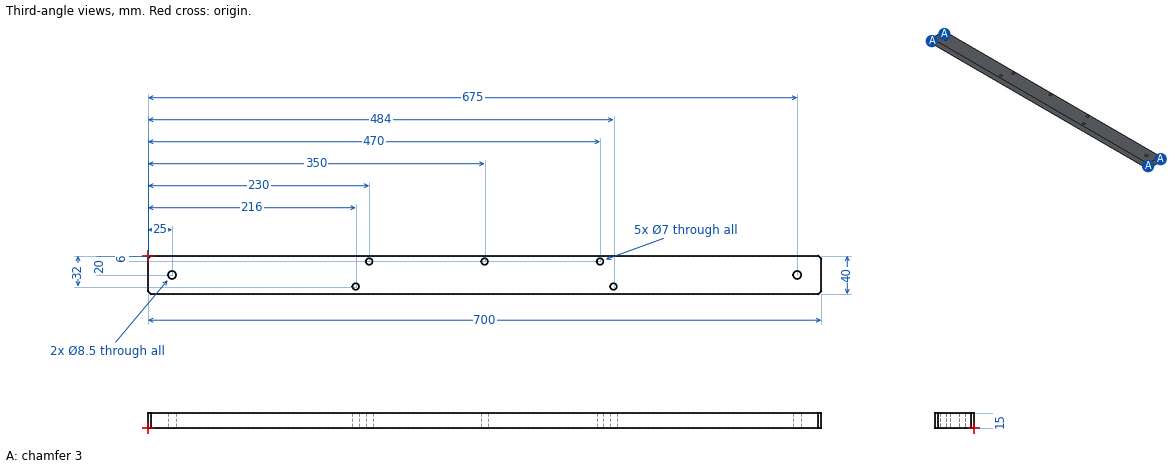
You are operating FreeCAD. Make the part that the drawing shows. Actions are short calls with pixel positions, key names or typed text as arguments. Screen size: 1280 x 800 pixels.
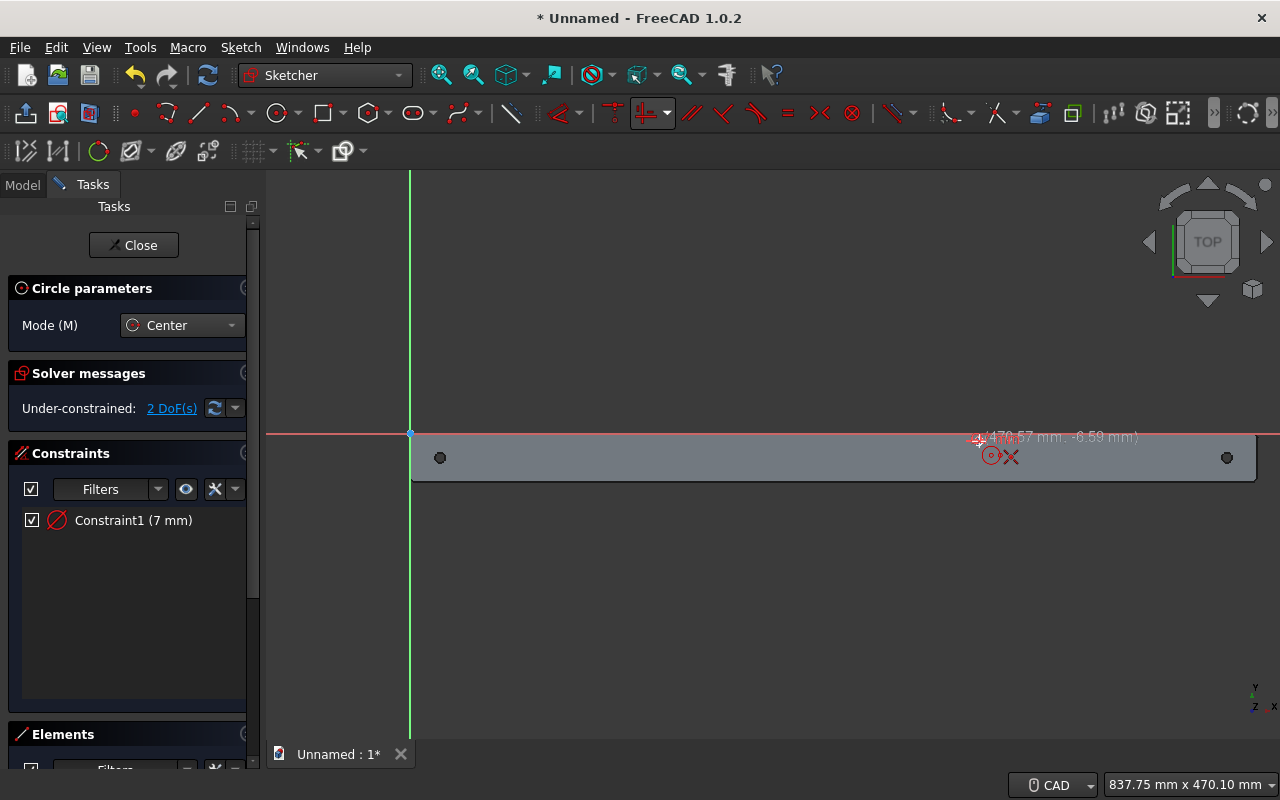
scroll(834, 441, up, 9)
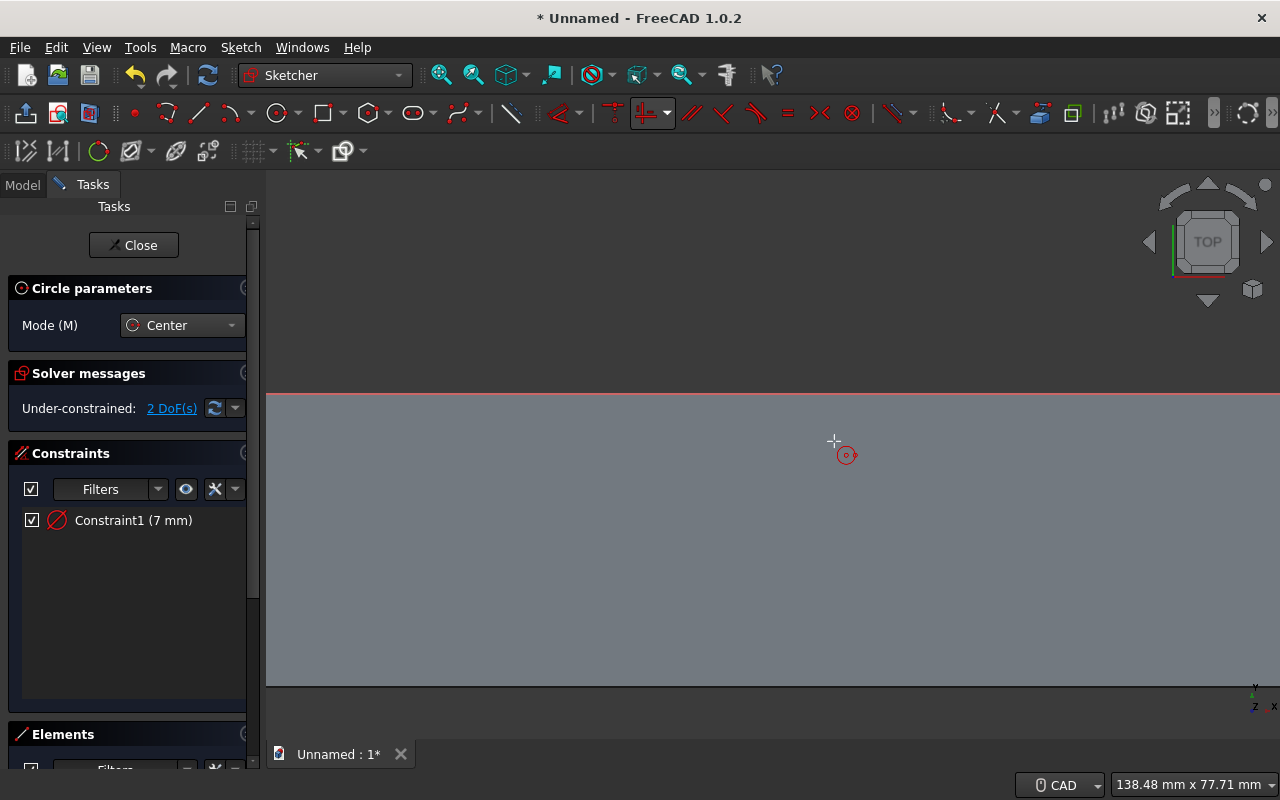
click(829, 438)
move(847, 420)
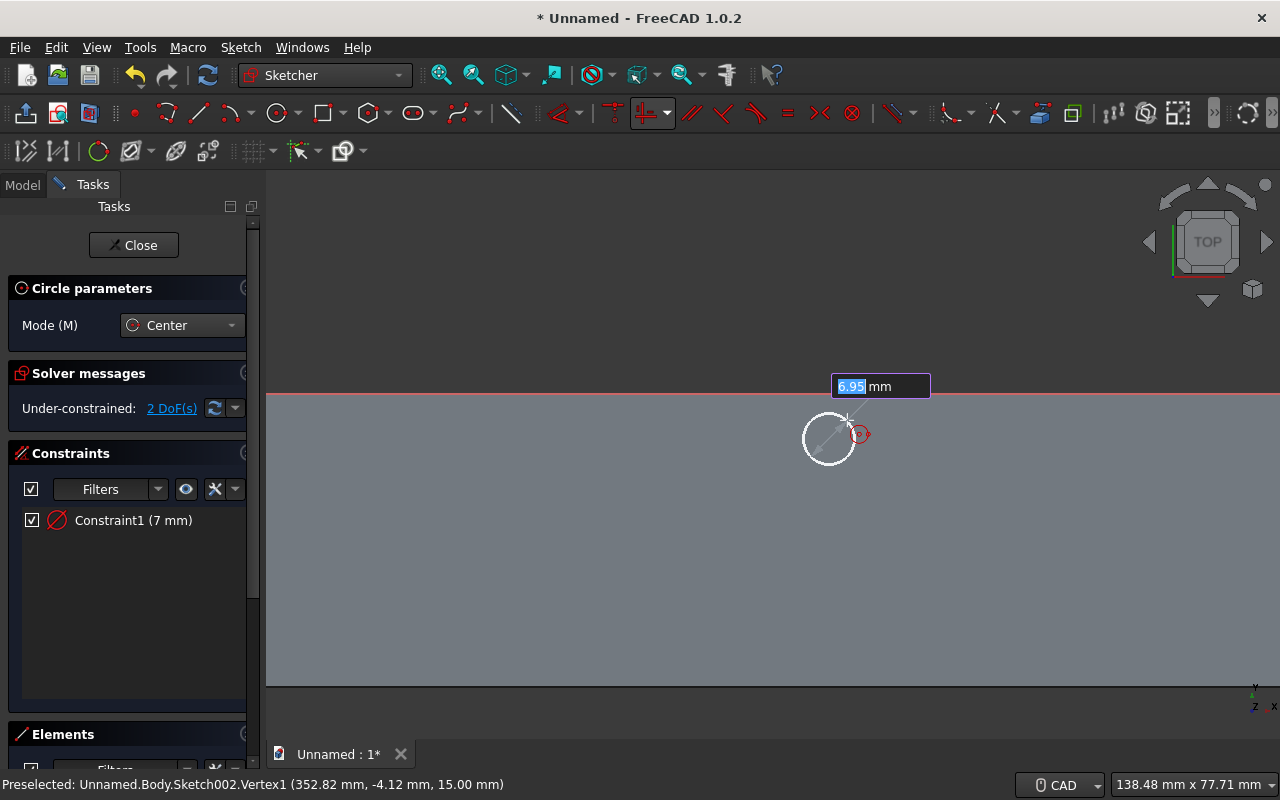
text(7)
key(Return)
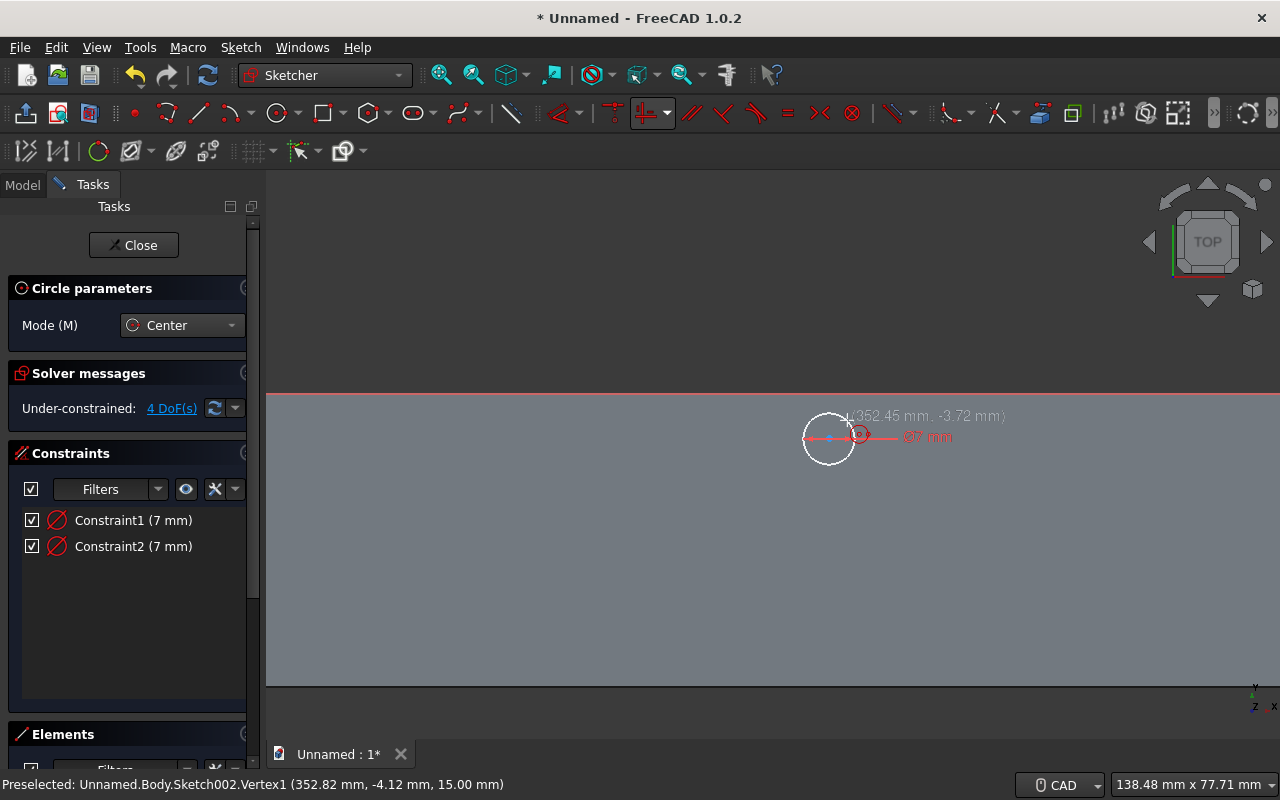
scroll(834, 441, down, 9)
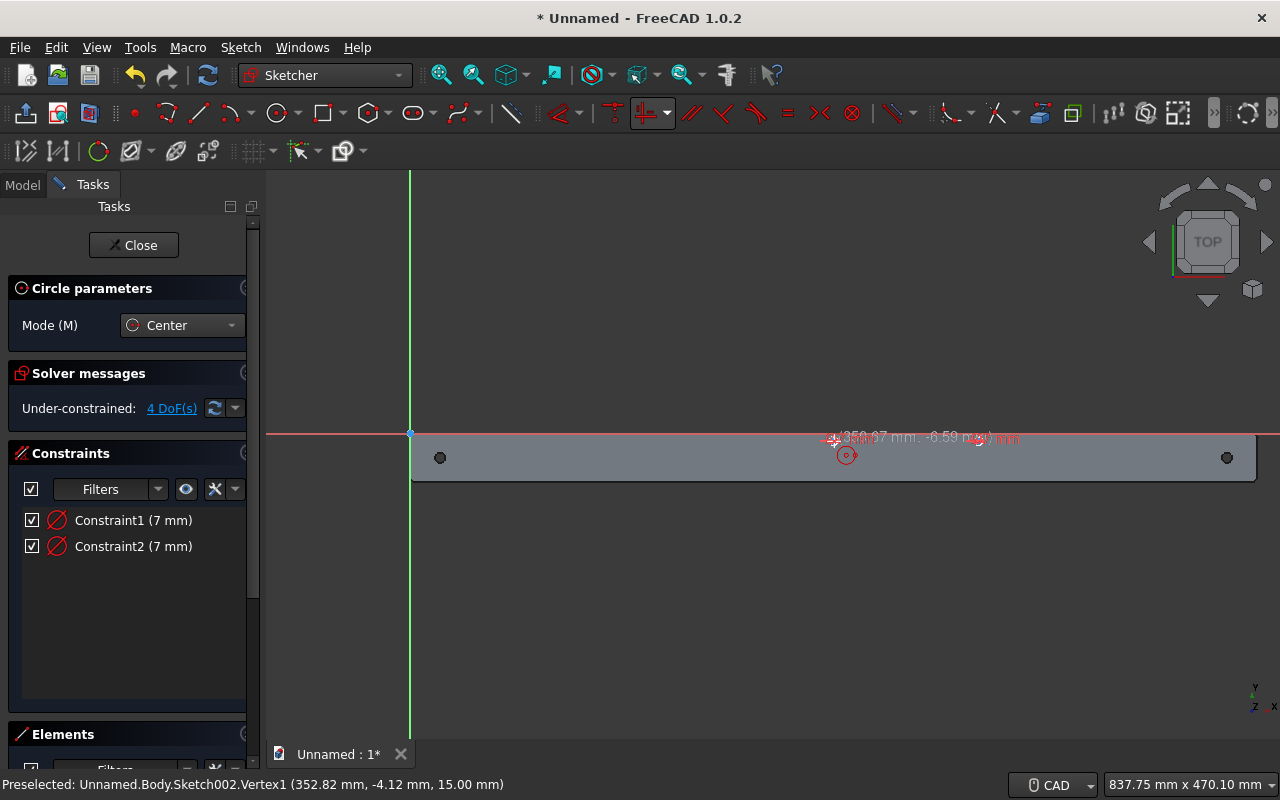
scroll(688, 441, up, 9)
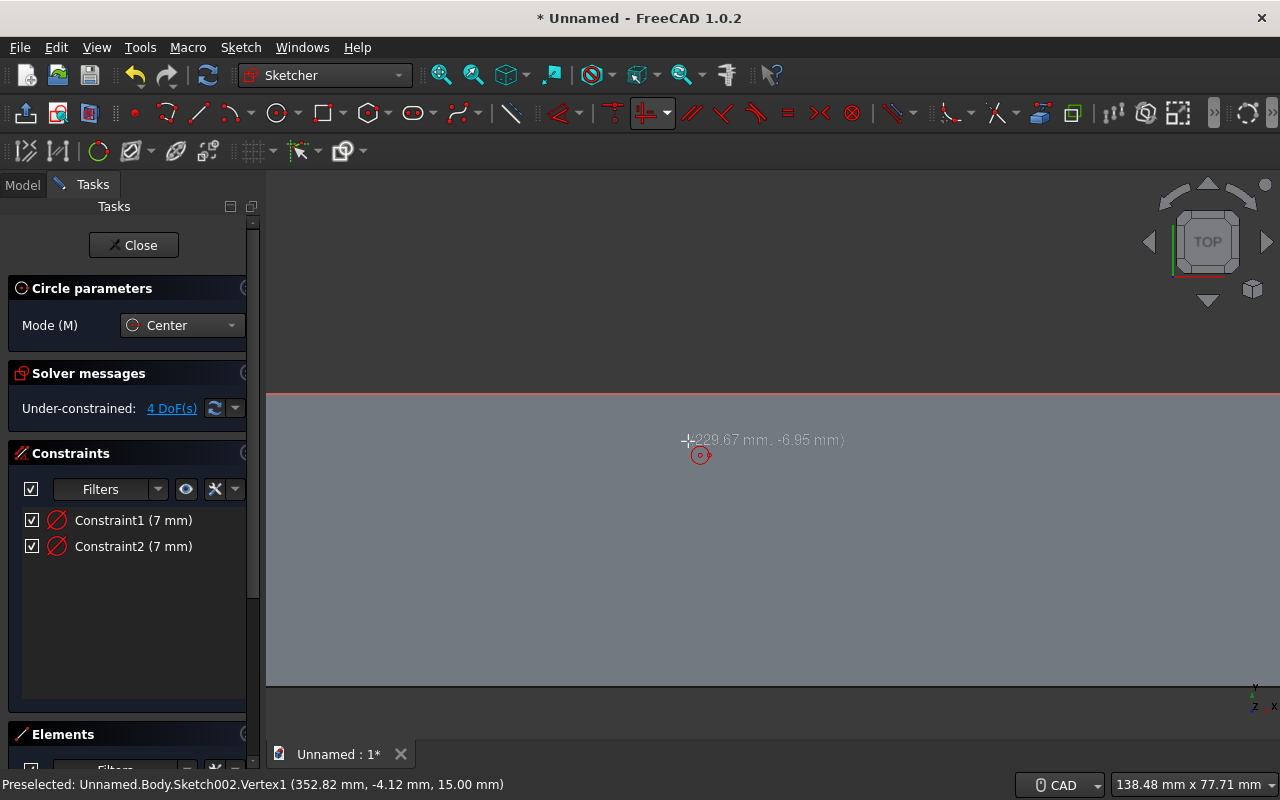
click(688, 438)
move(706, 420)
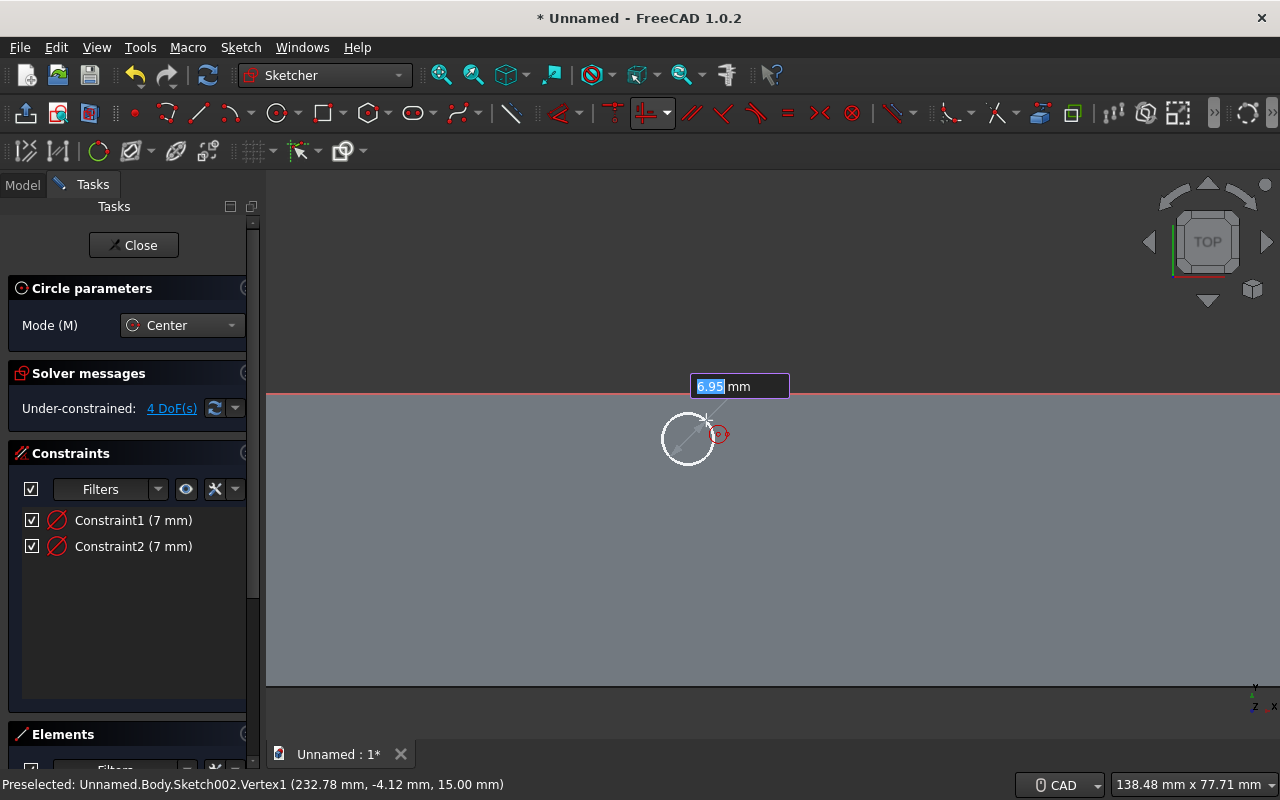
text(7)
key(Return)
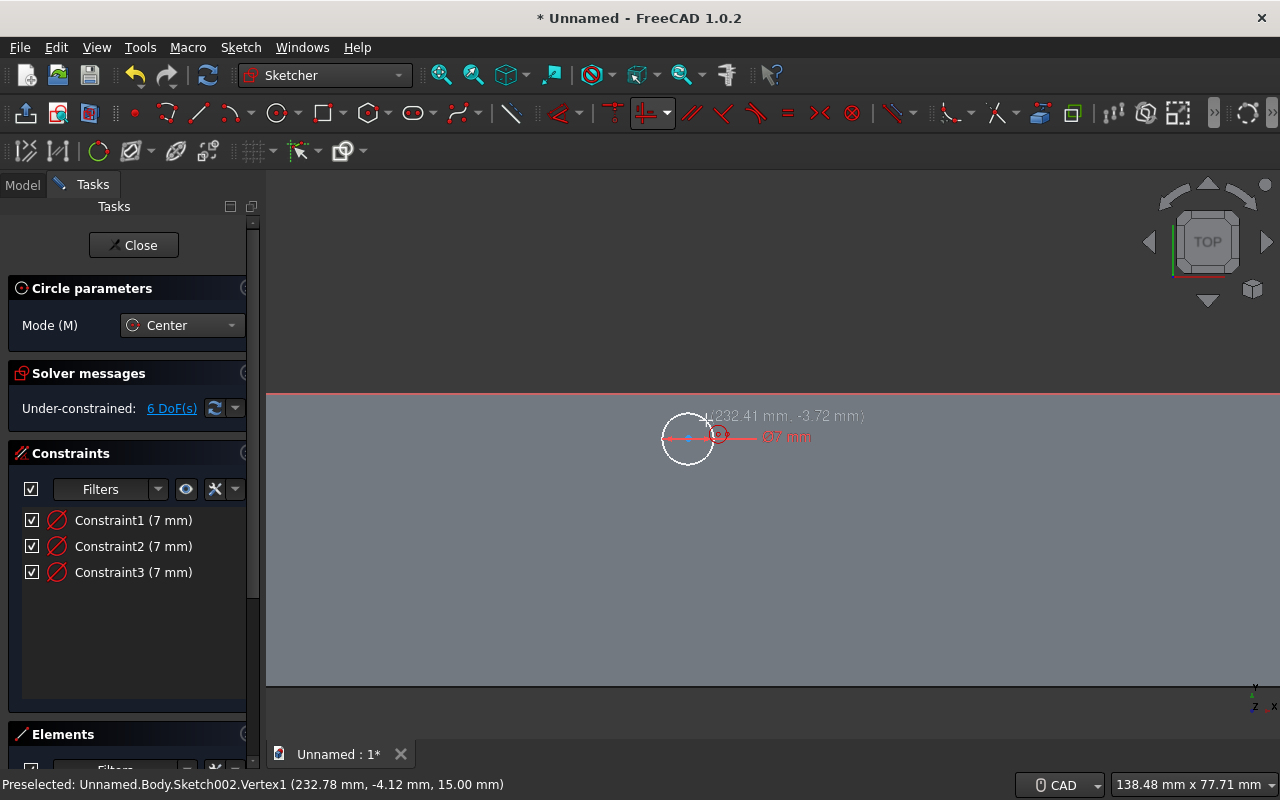
scroll(688, 441, down, 9)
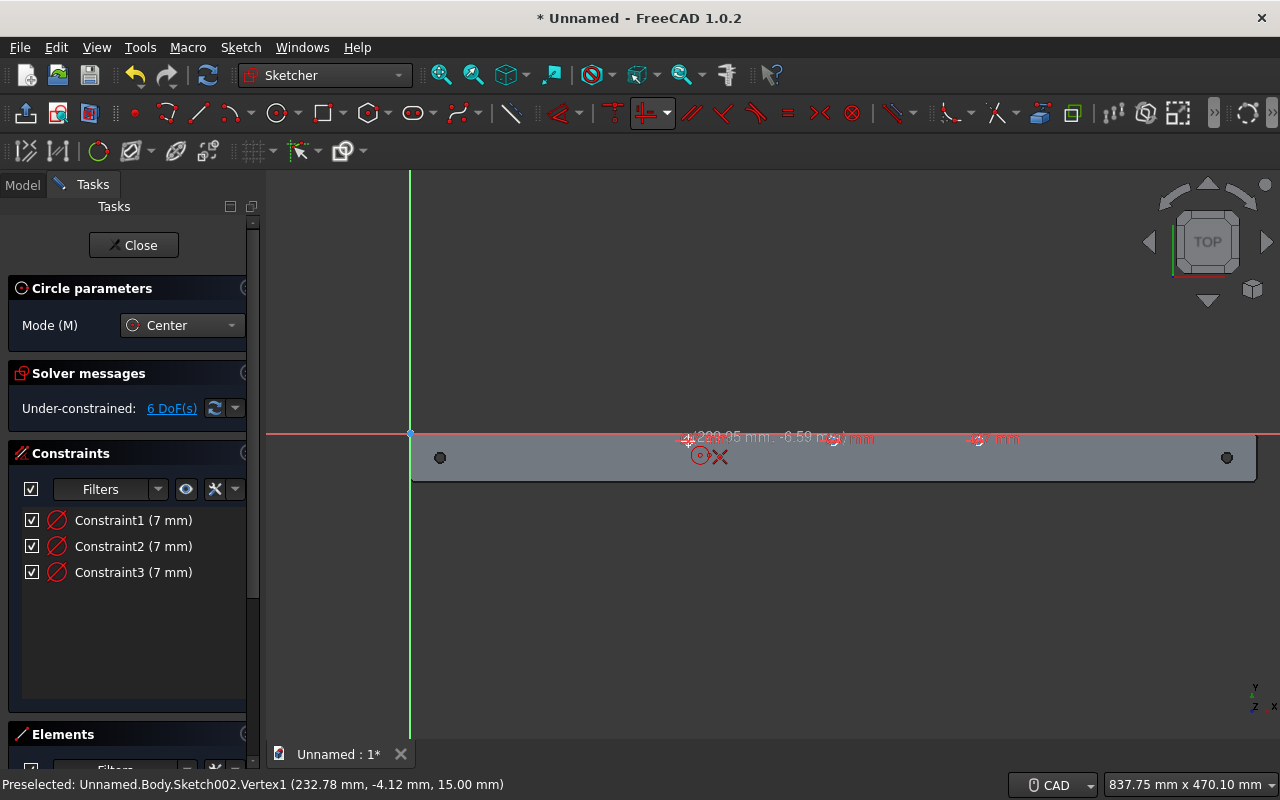
click(671, 472)
move(674, 469)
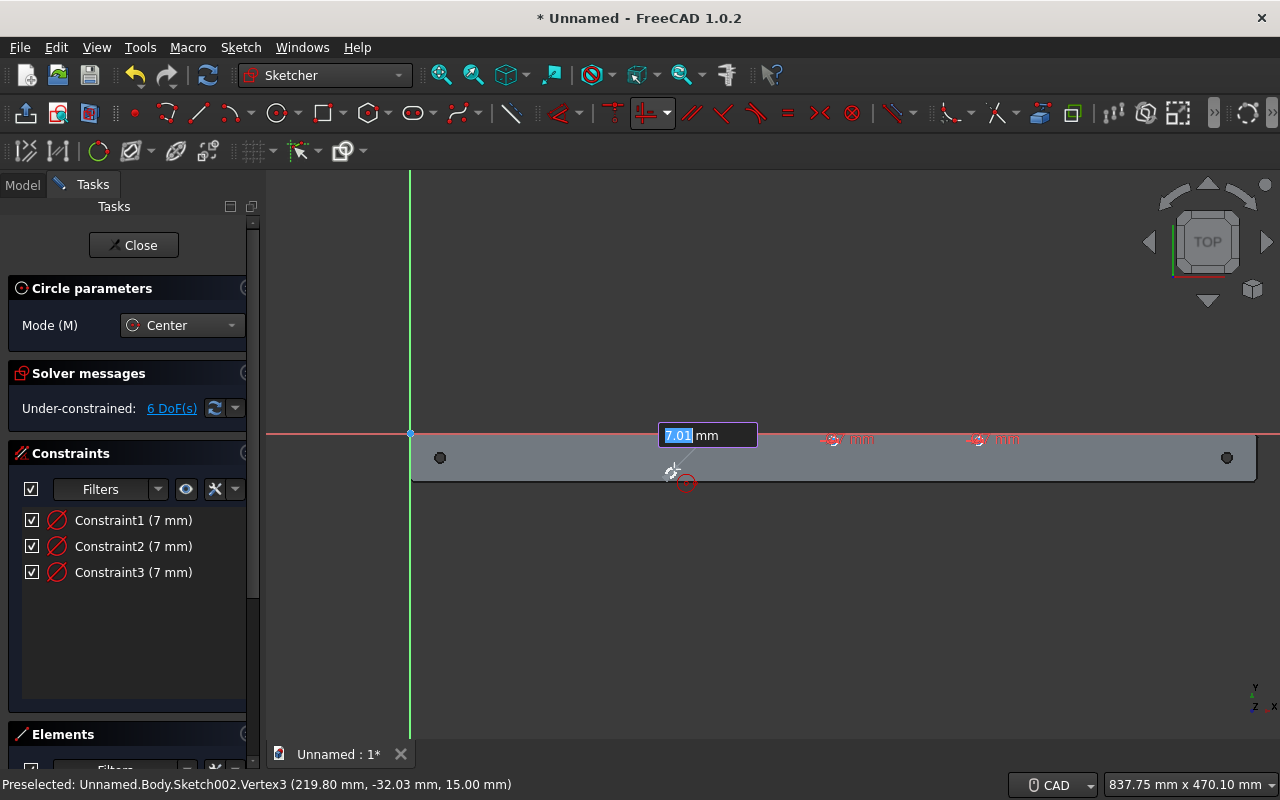
text(7)
key(Return)